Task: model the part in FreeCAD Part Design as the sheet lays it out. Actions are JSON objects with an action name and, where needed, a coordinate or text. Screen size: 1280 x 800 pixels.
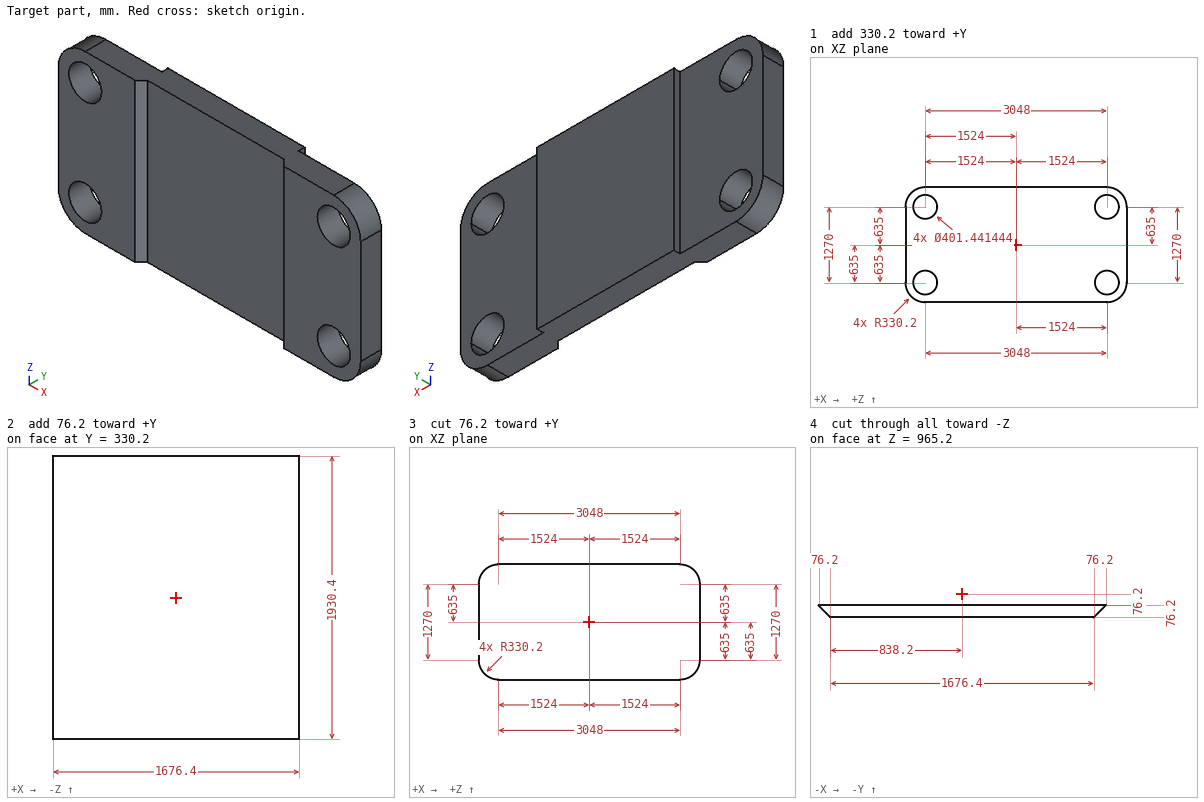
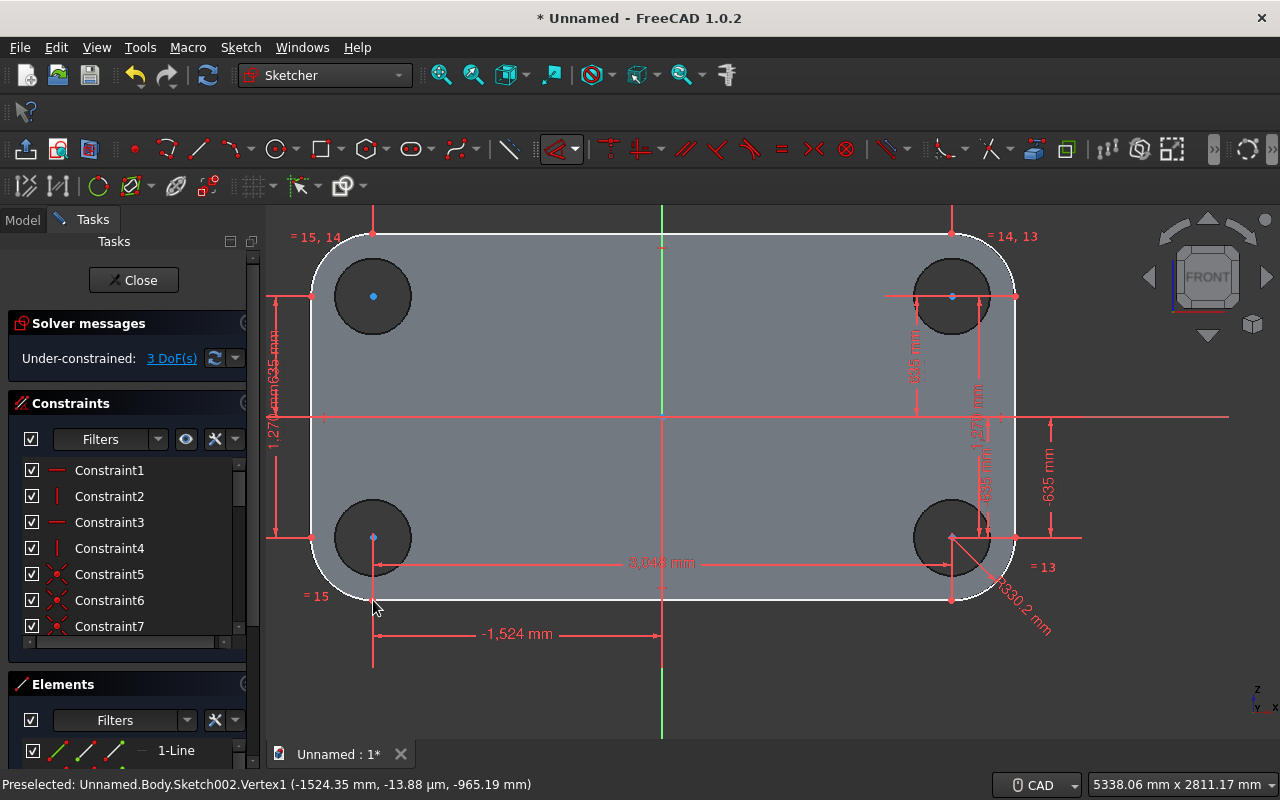
{"action": "left_click", "coordinate": [952, 234]}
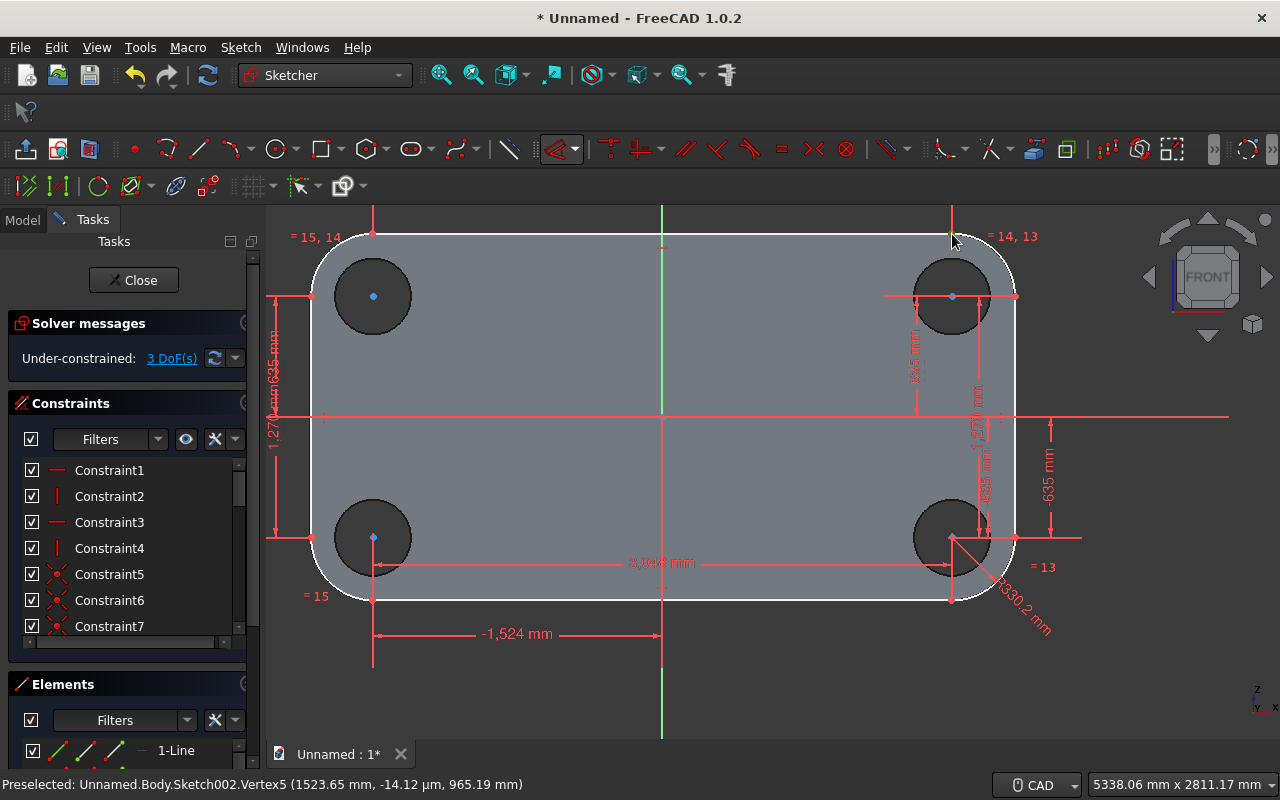
{"action": "key", "text": "l"}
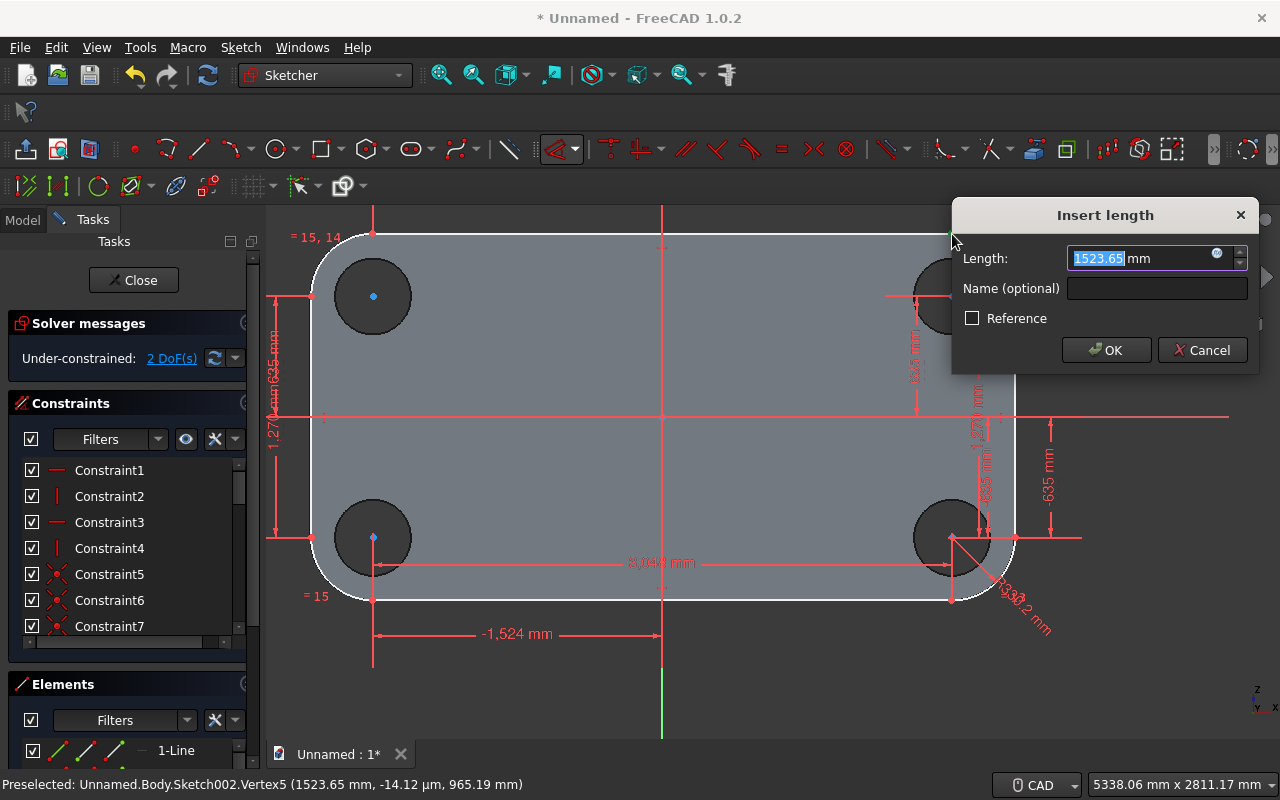
{"action": "type", "text": "1524"}
{"action": "key", "text": "Return"}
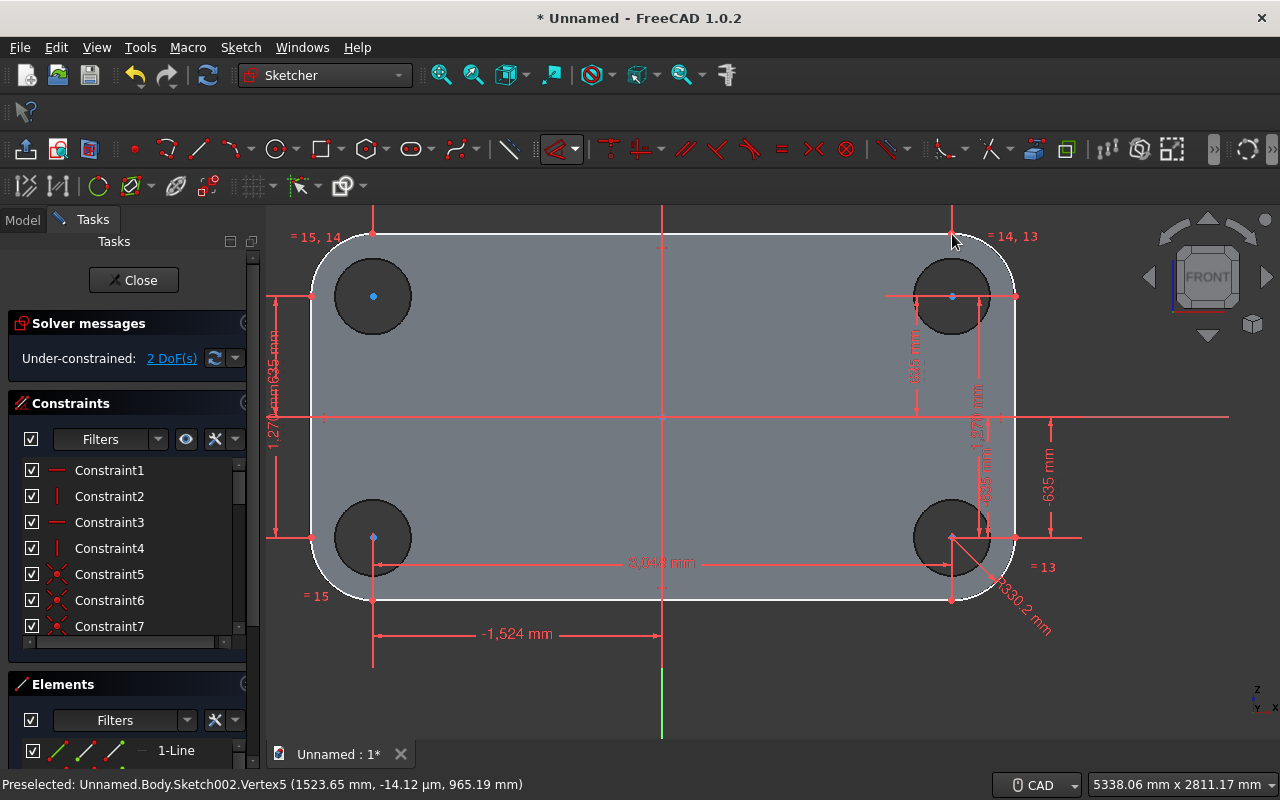
{"action": "left_click", "coordinate": [952, 538]}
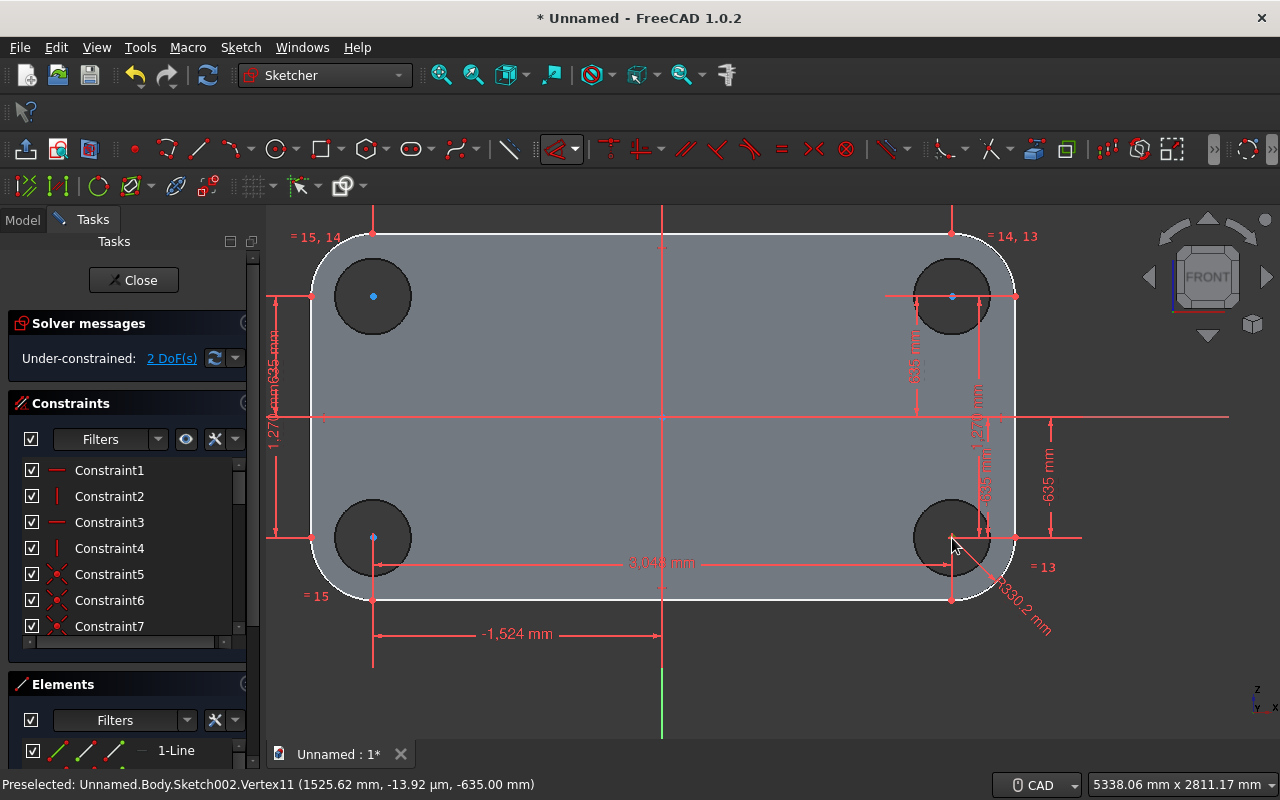
{"action": "left_click", "coordinate": [578, 150]}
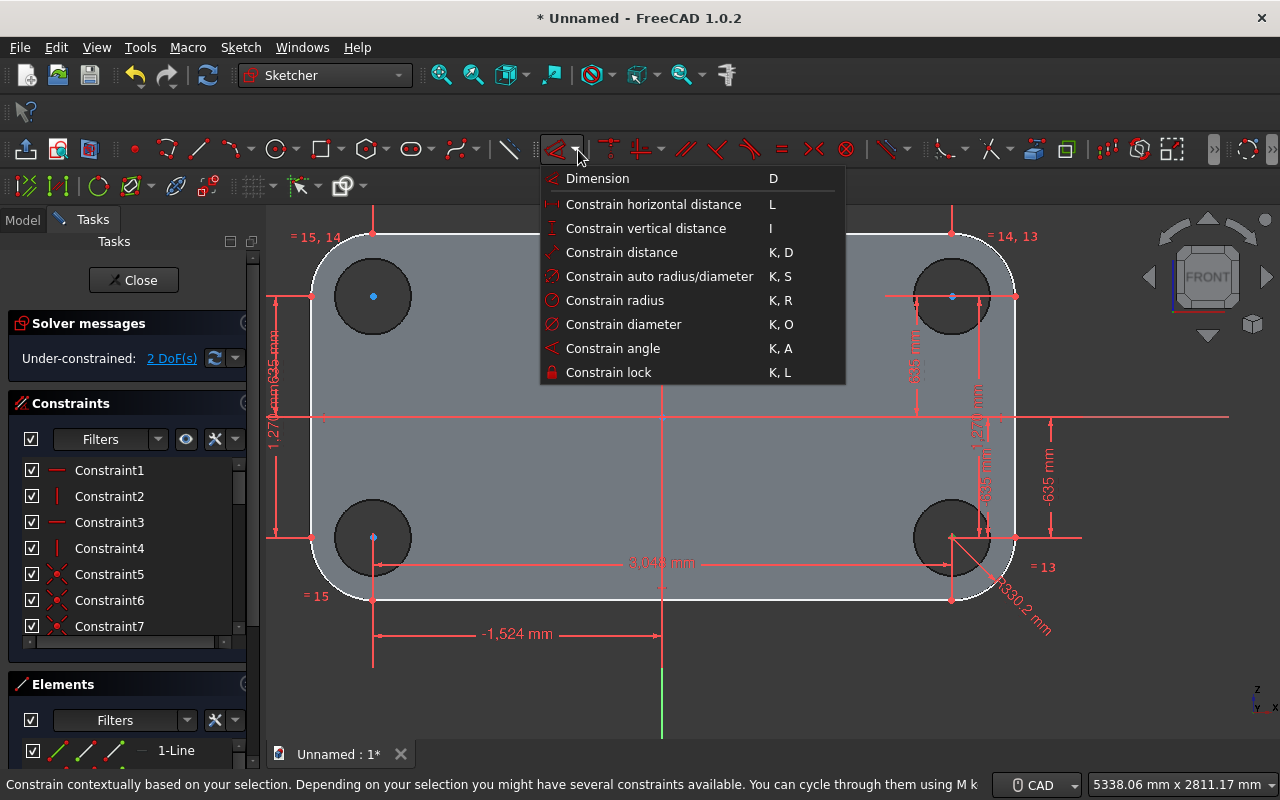
{"action": "left_click", "coordinate": [693, 204]}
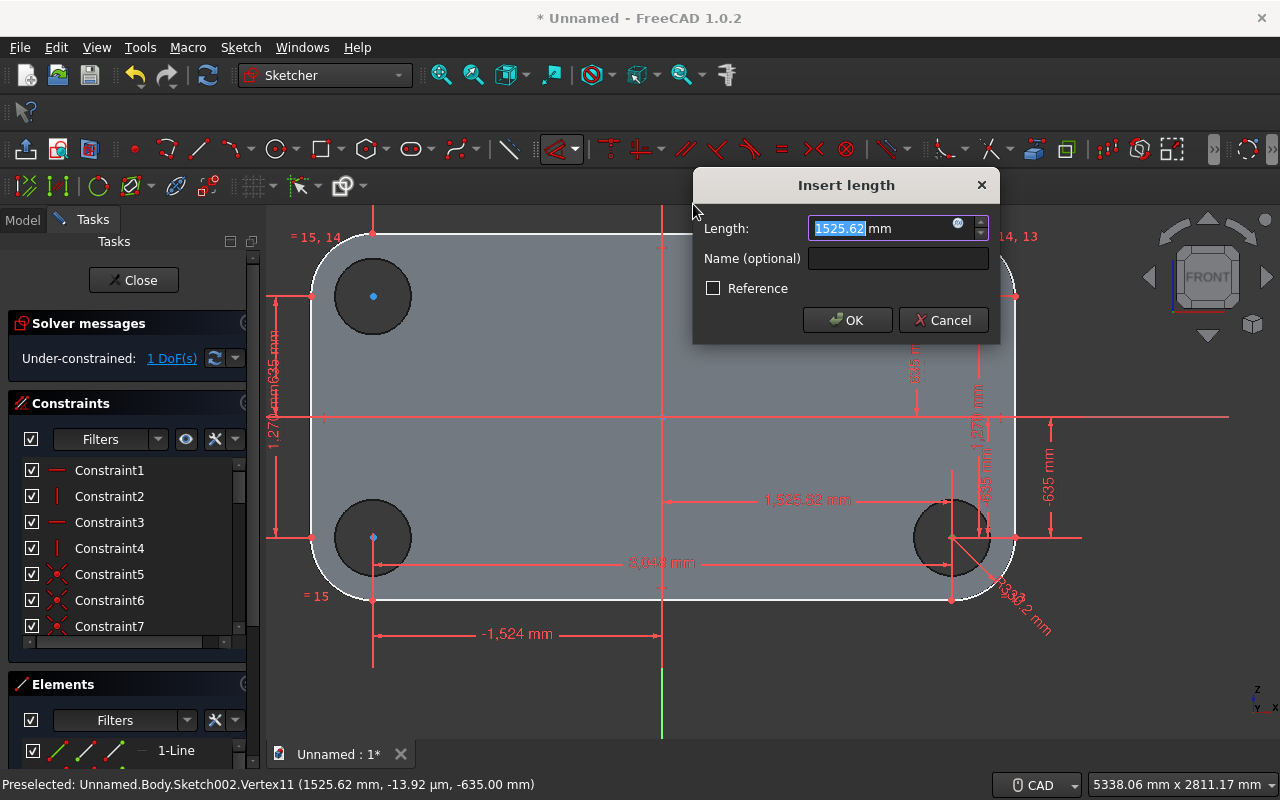
{"action": "type", "text": "1524"}
{"action": "key", "text": "Return"}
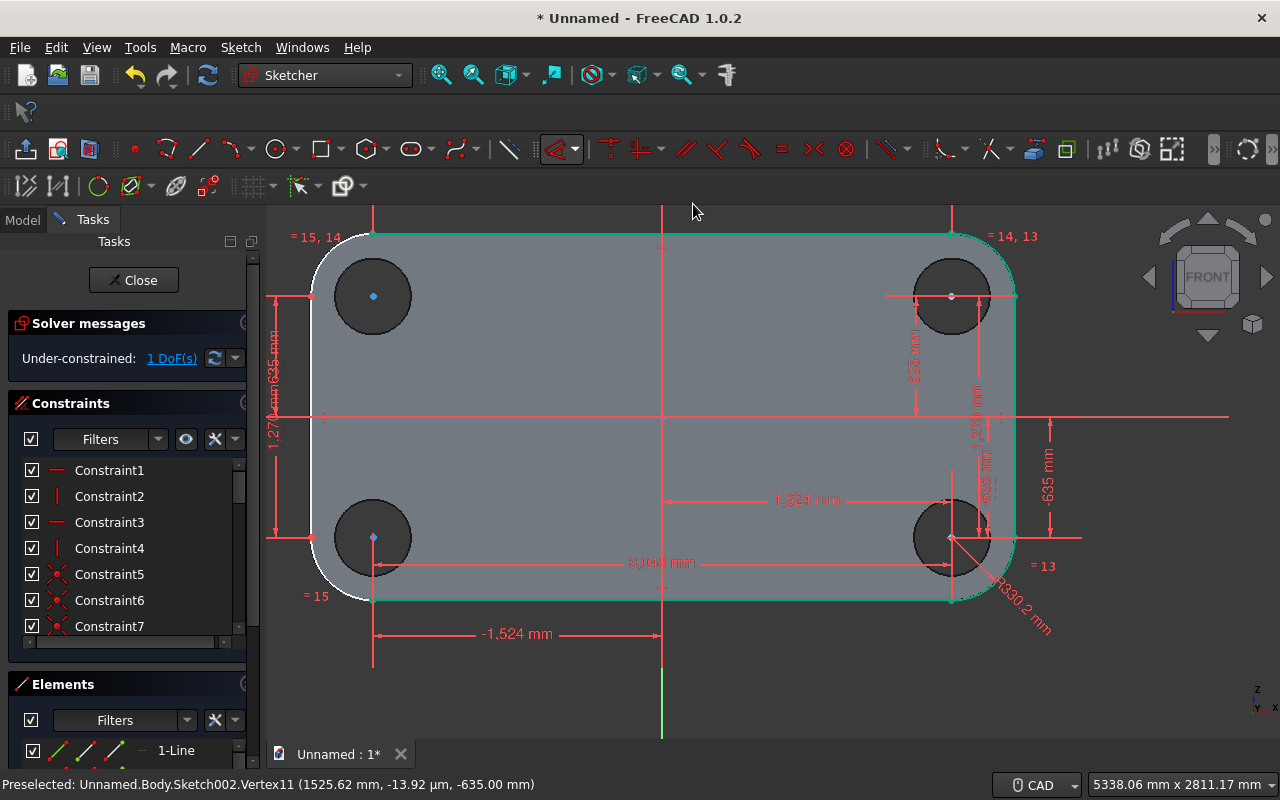
{"action": "left_click", "coordinate": [374, 296]}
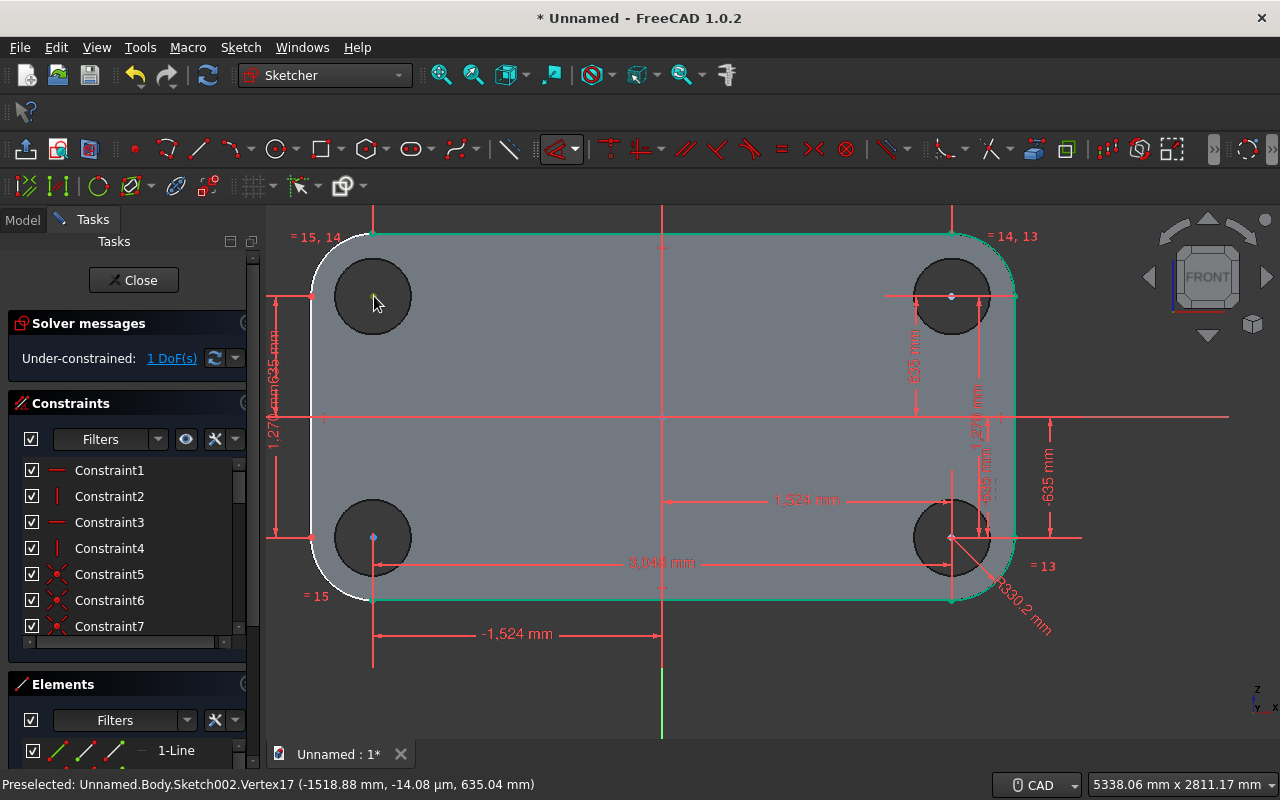
{"action": "key", "text": "l"}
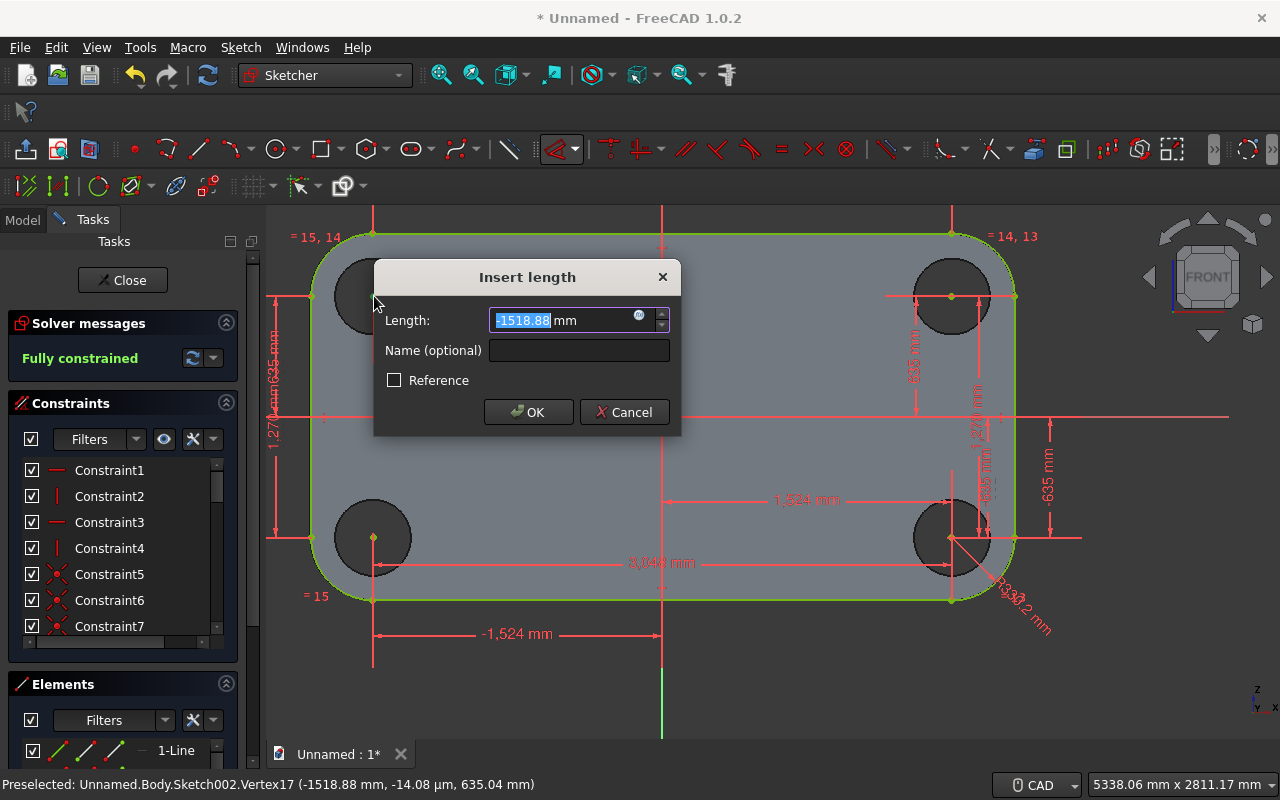
{"action": "type", "text": "-1524"}
{"action": "key", "text": "Return"}